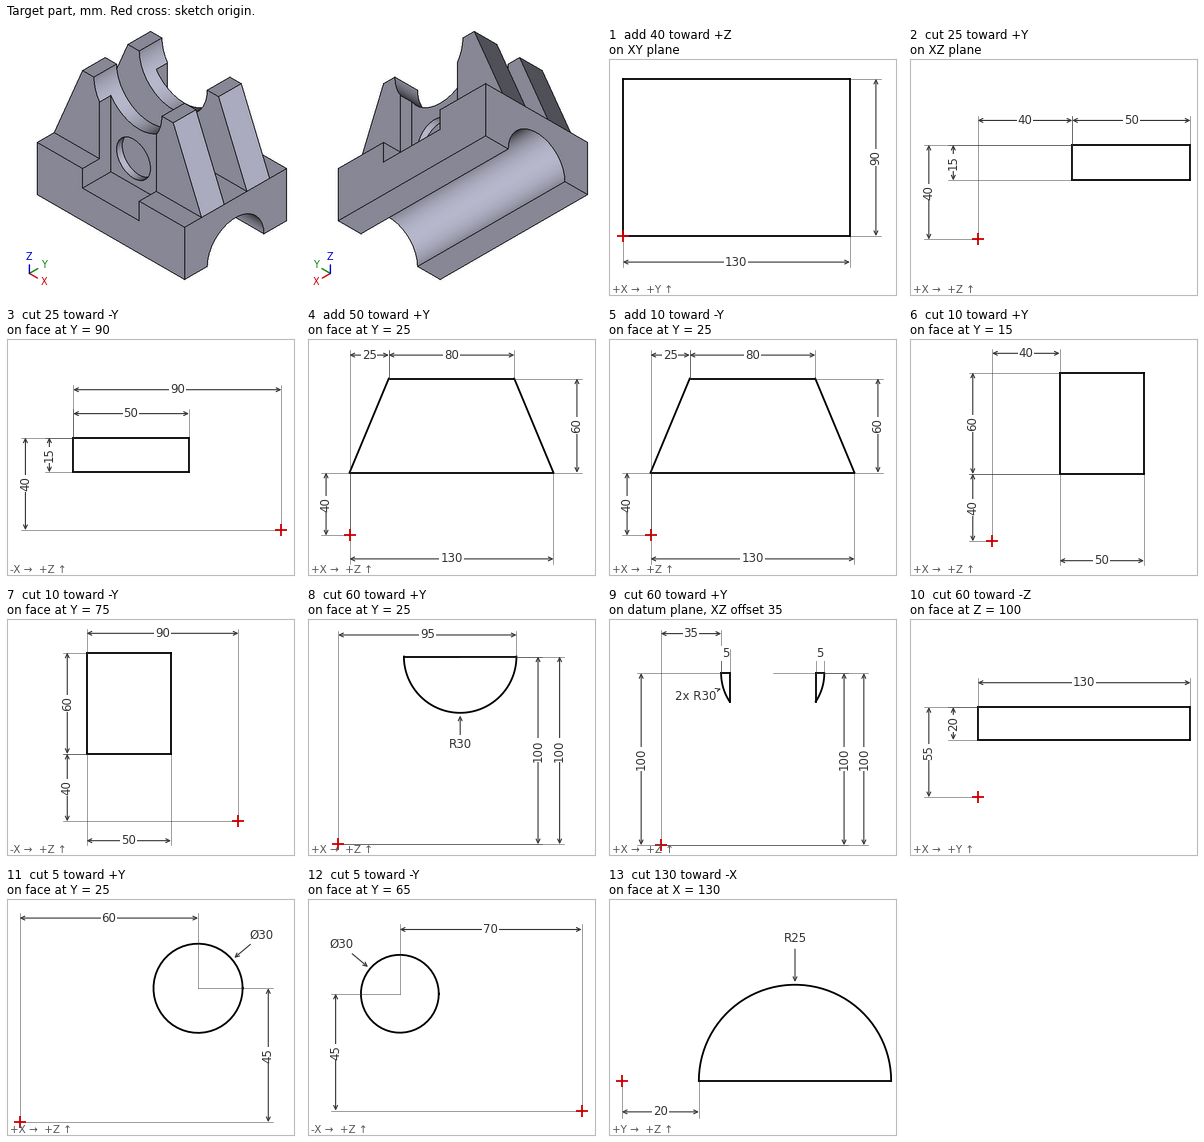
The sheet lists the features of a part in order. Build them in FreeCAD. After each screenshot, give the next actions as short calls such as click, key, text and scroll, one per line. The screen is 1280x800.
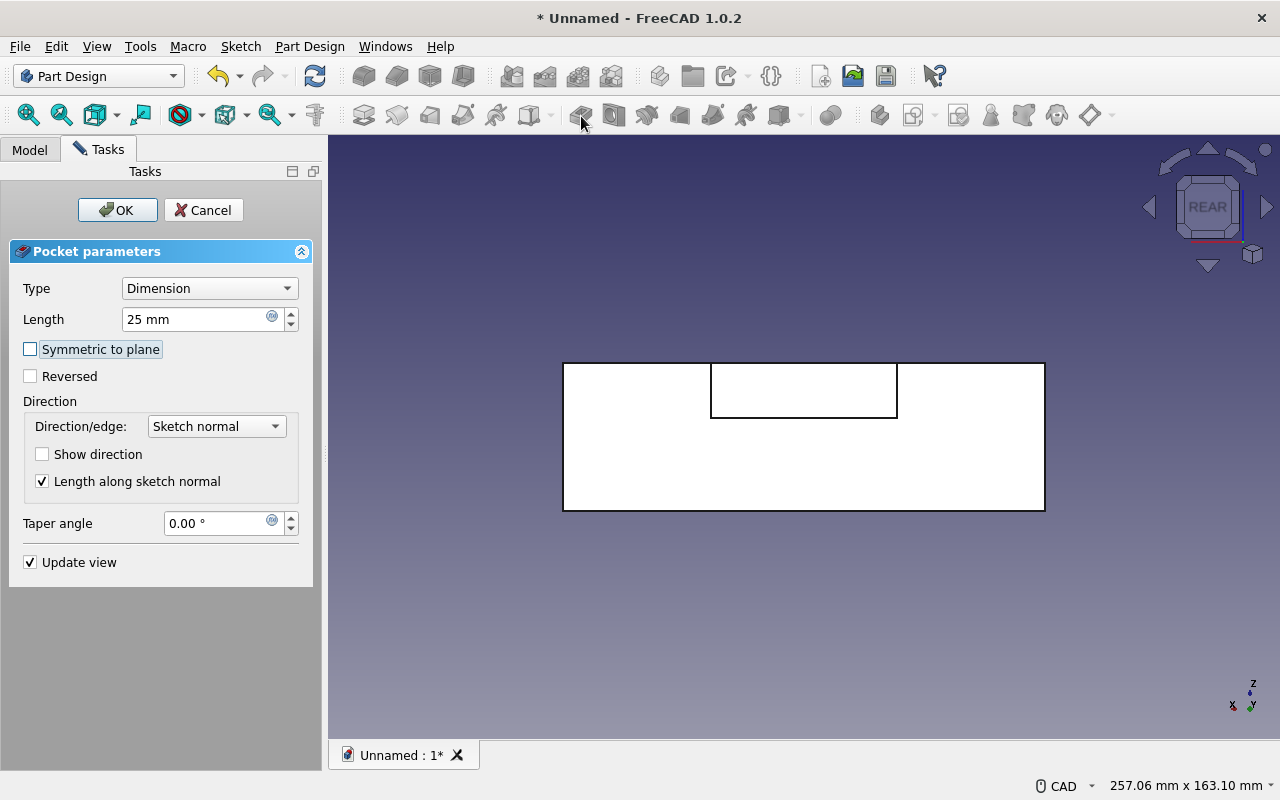
click(118, 210)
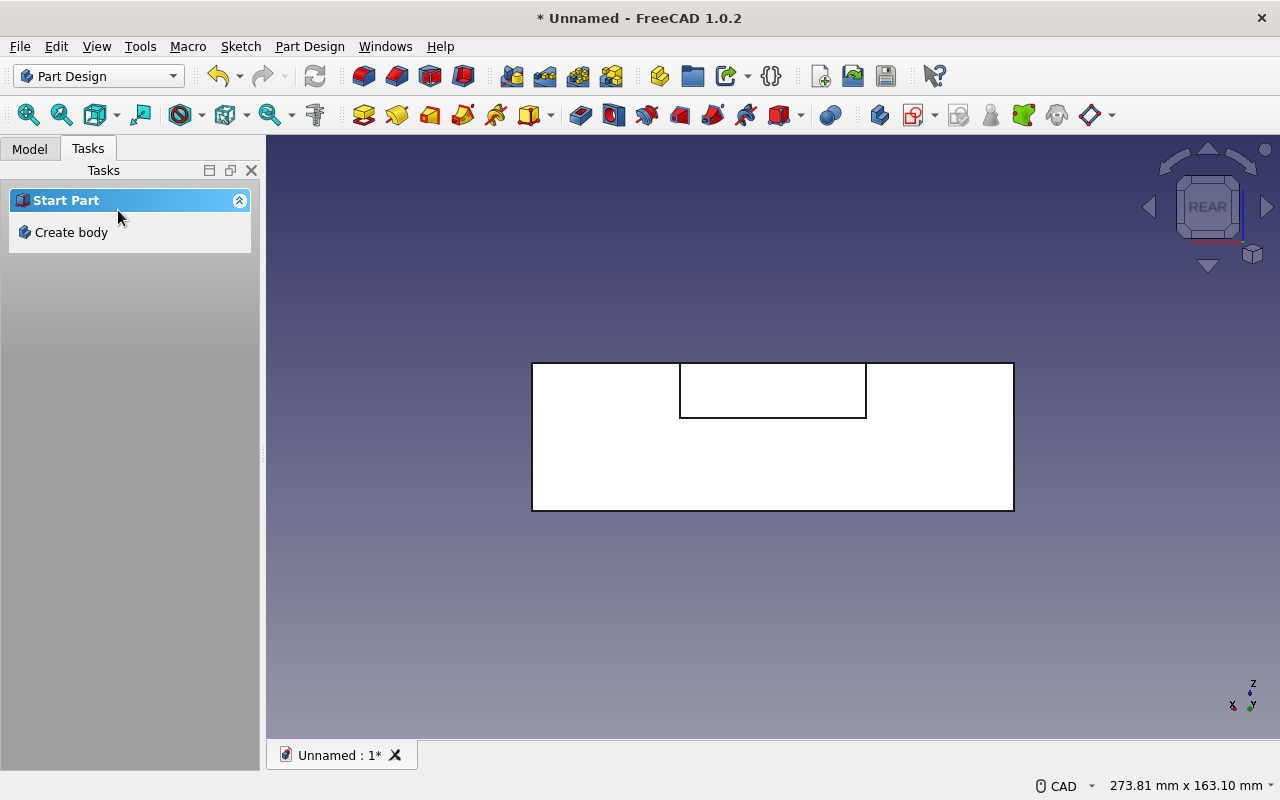
key(0)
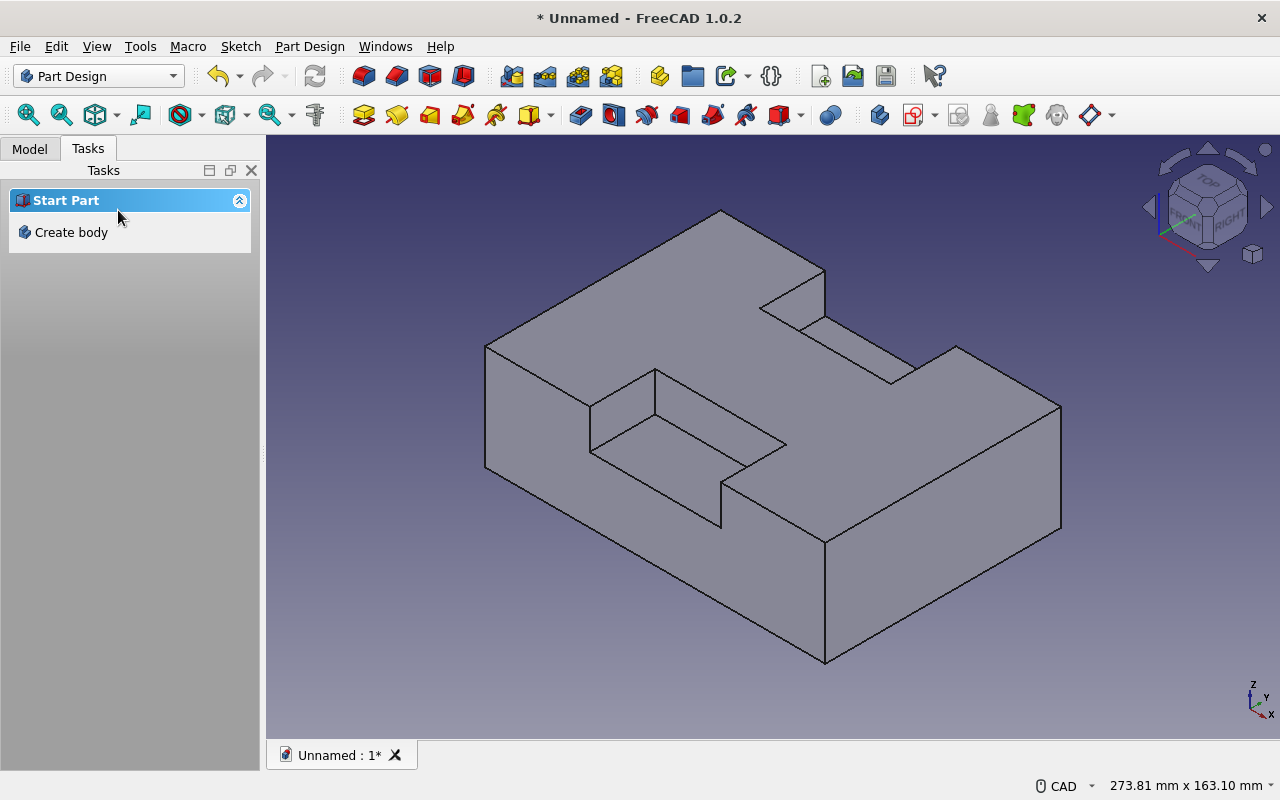
click(739, 439)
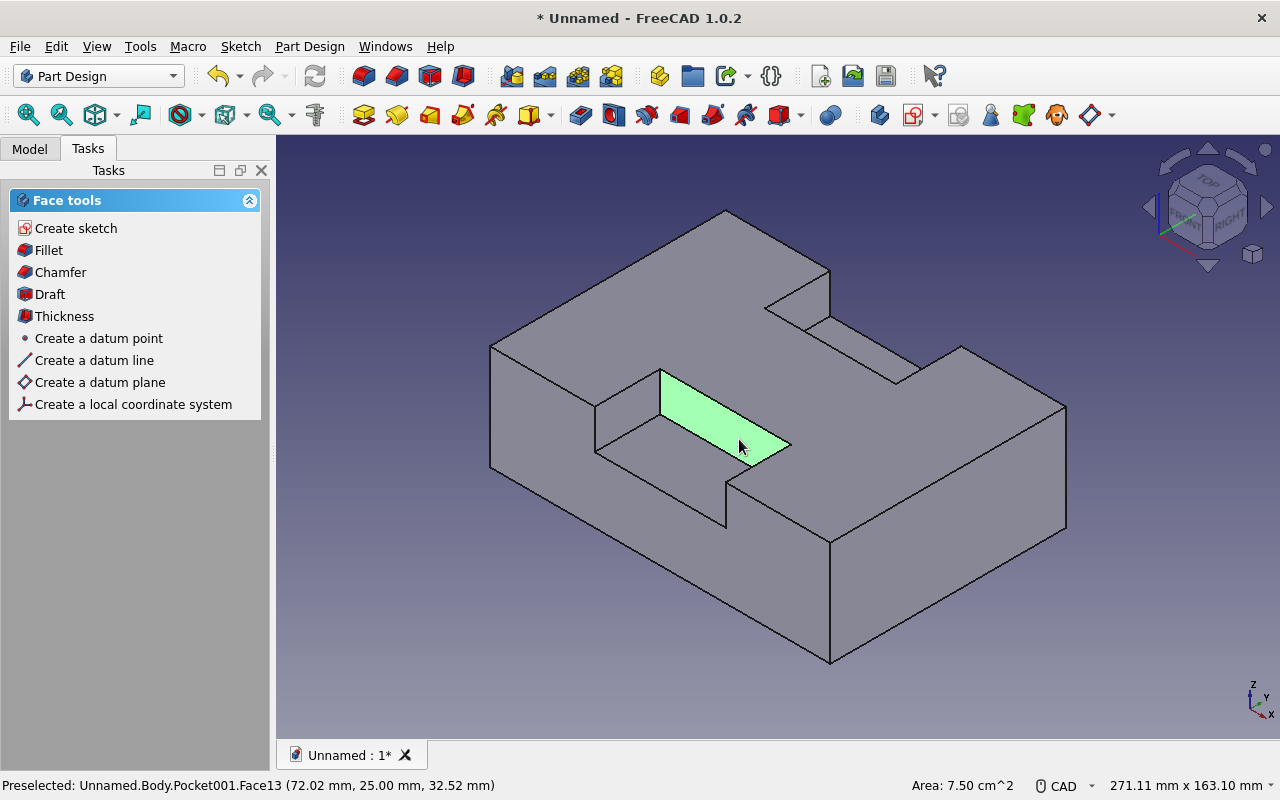
click(912, 116)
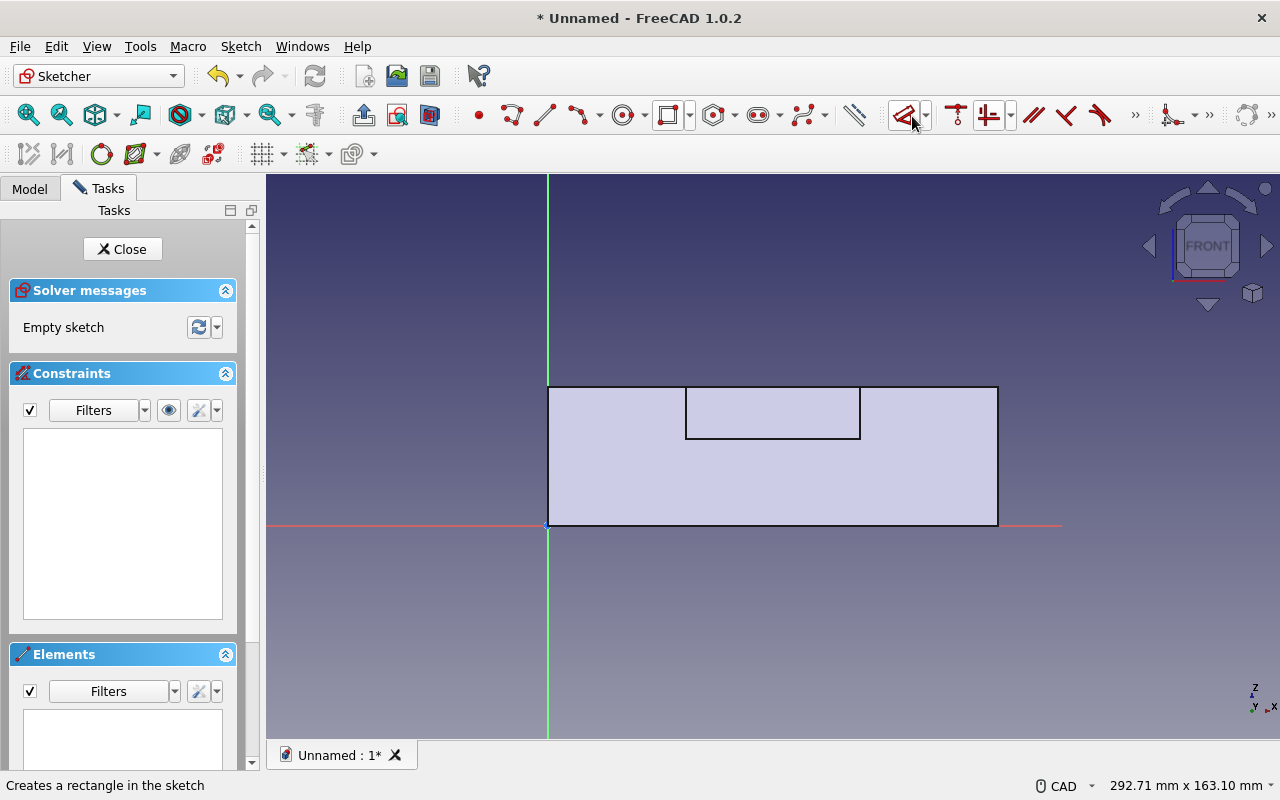
key(q)
key(s)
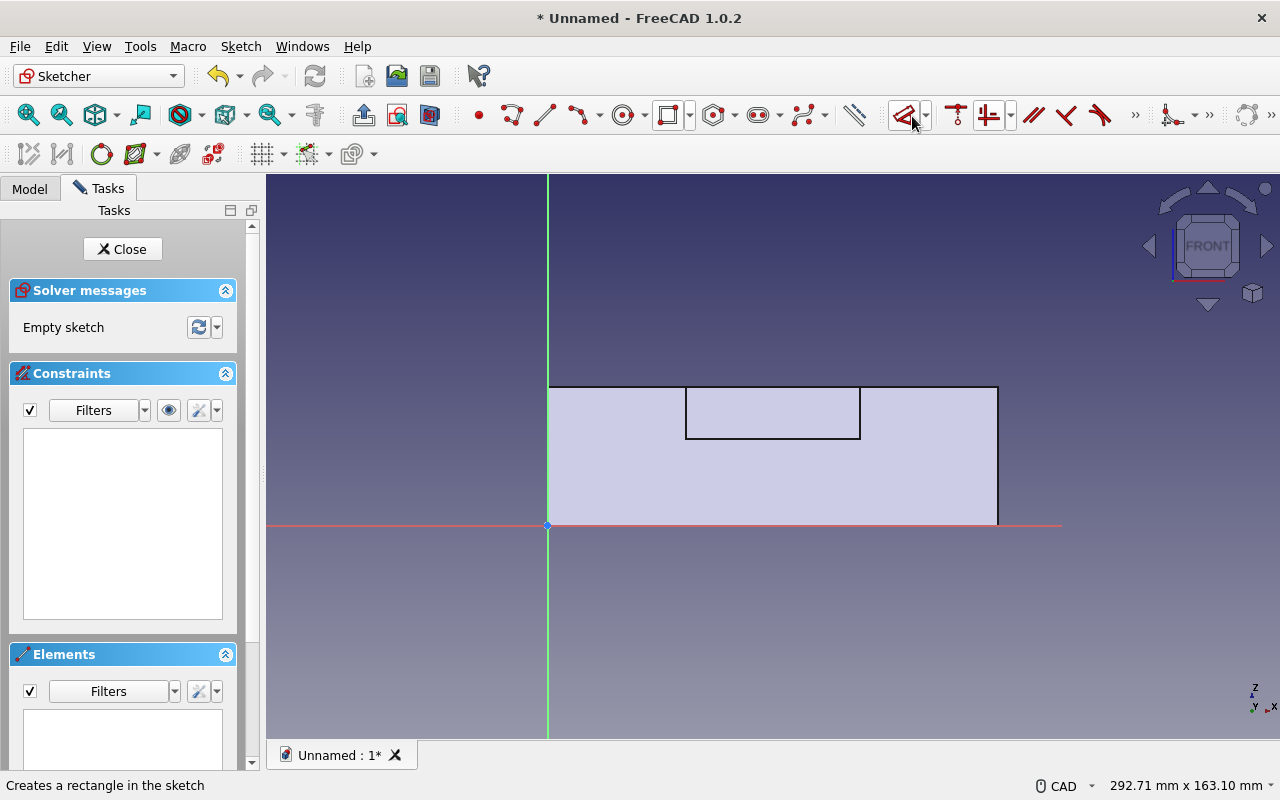
scroll(395, 711, down, 1)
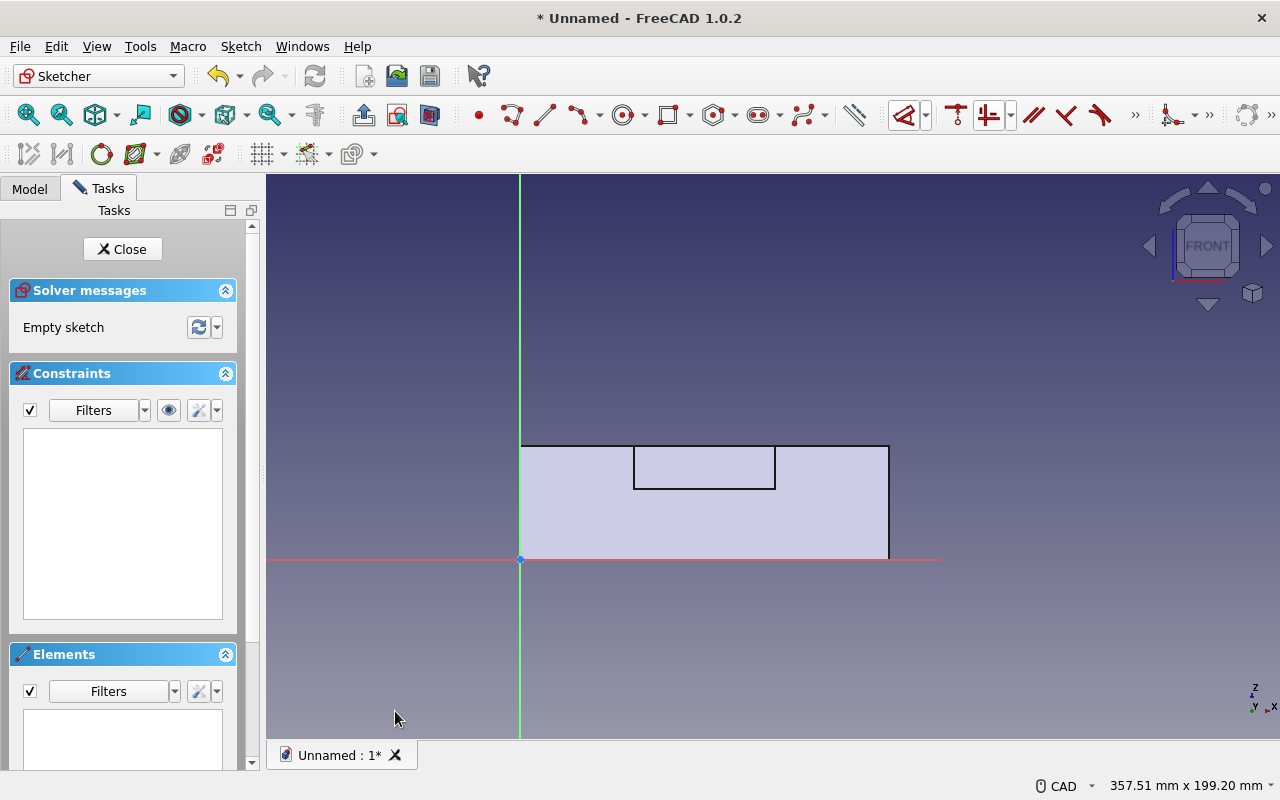
click(512, 116)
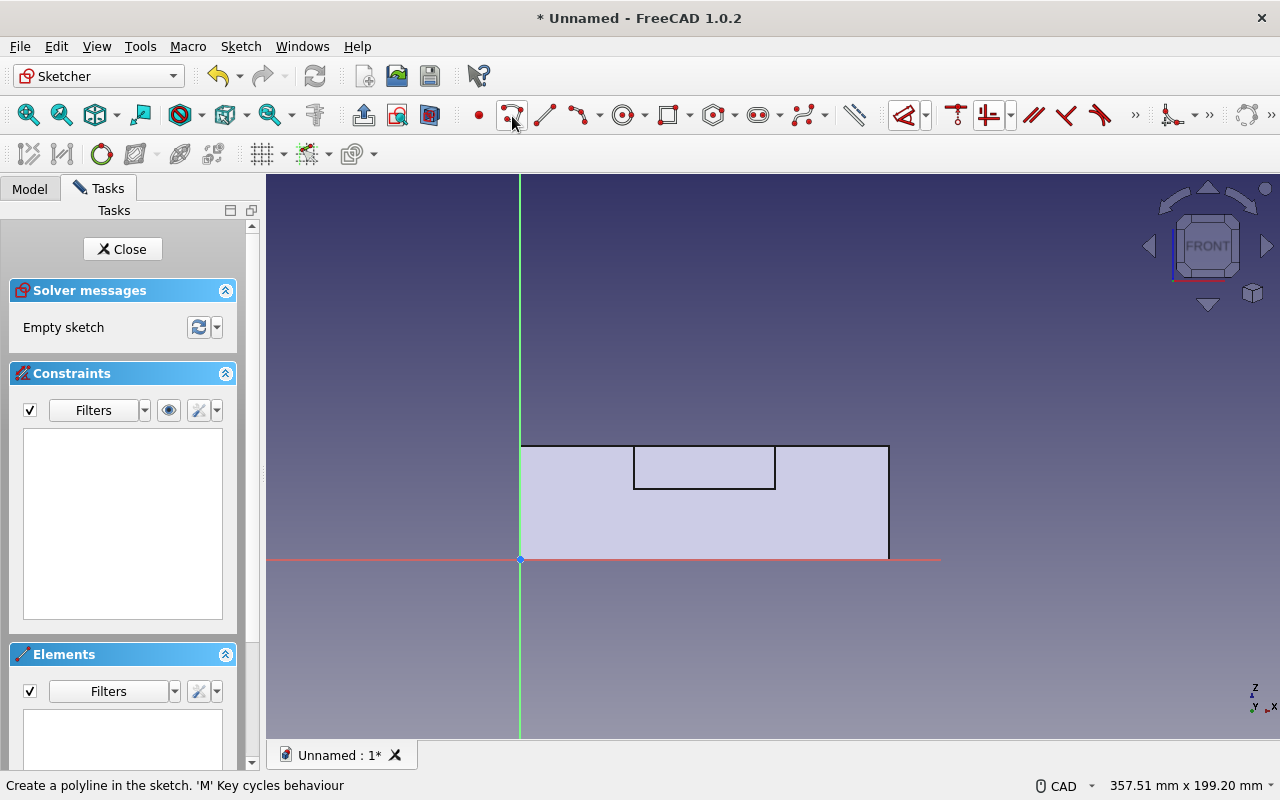
click(520, 446)
click(889, 446)
click(818, 276)
click(591, 276)
click(520, 447)
key(Escape)
key(Escape)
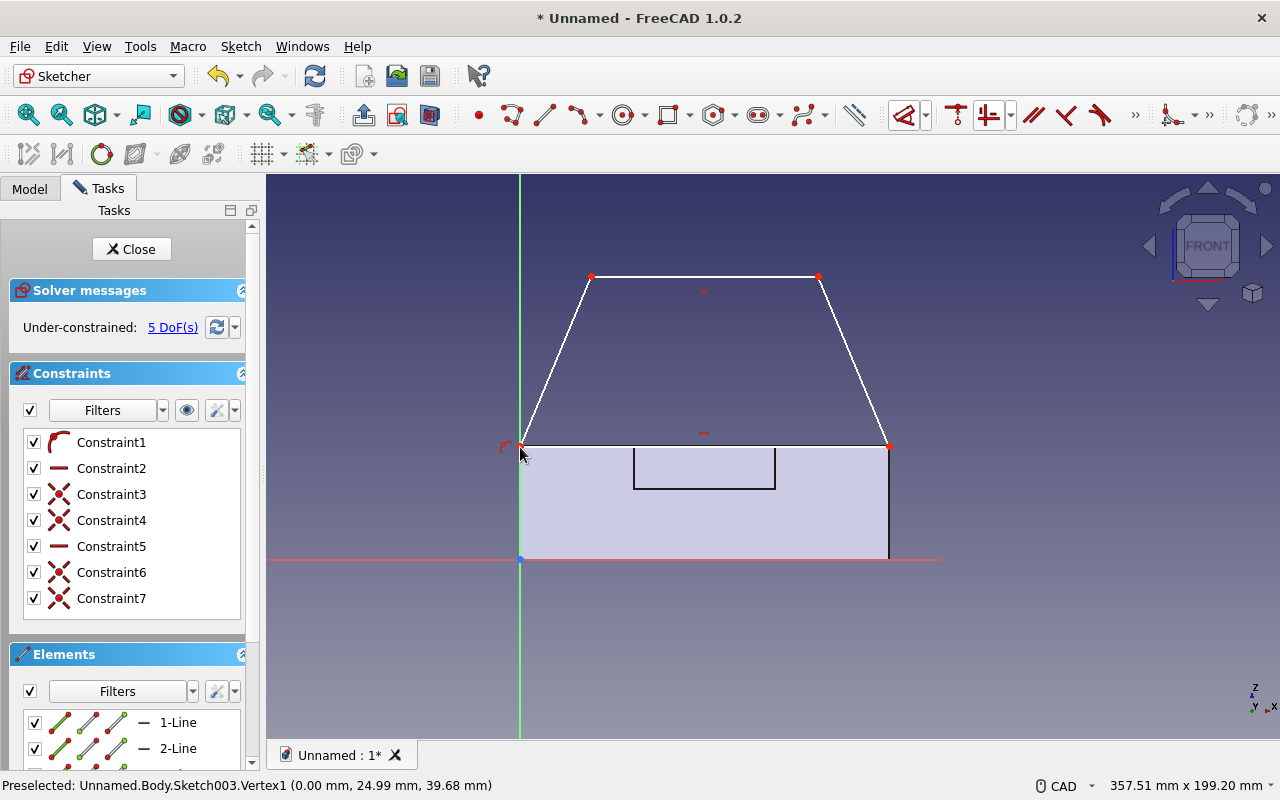
key(d)